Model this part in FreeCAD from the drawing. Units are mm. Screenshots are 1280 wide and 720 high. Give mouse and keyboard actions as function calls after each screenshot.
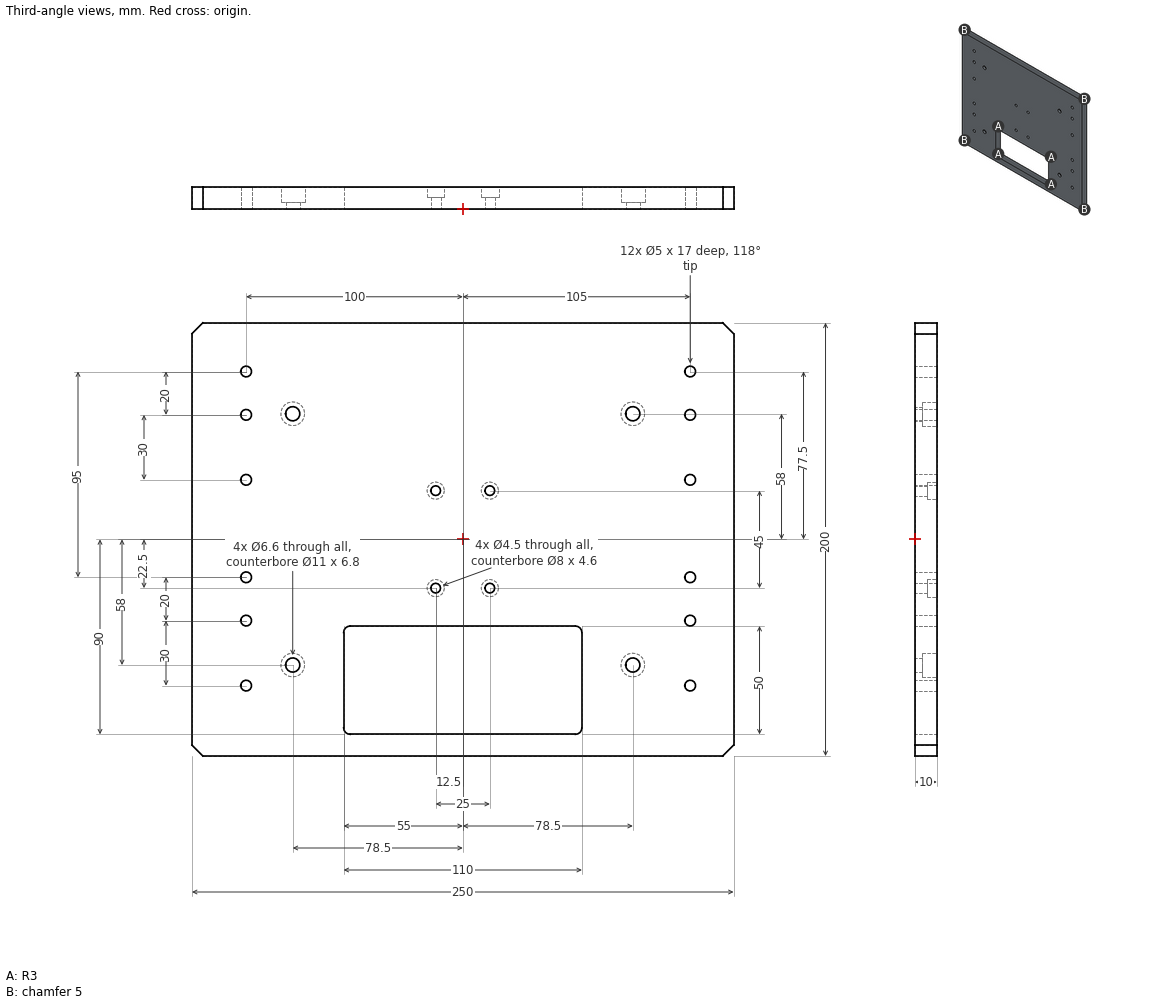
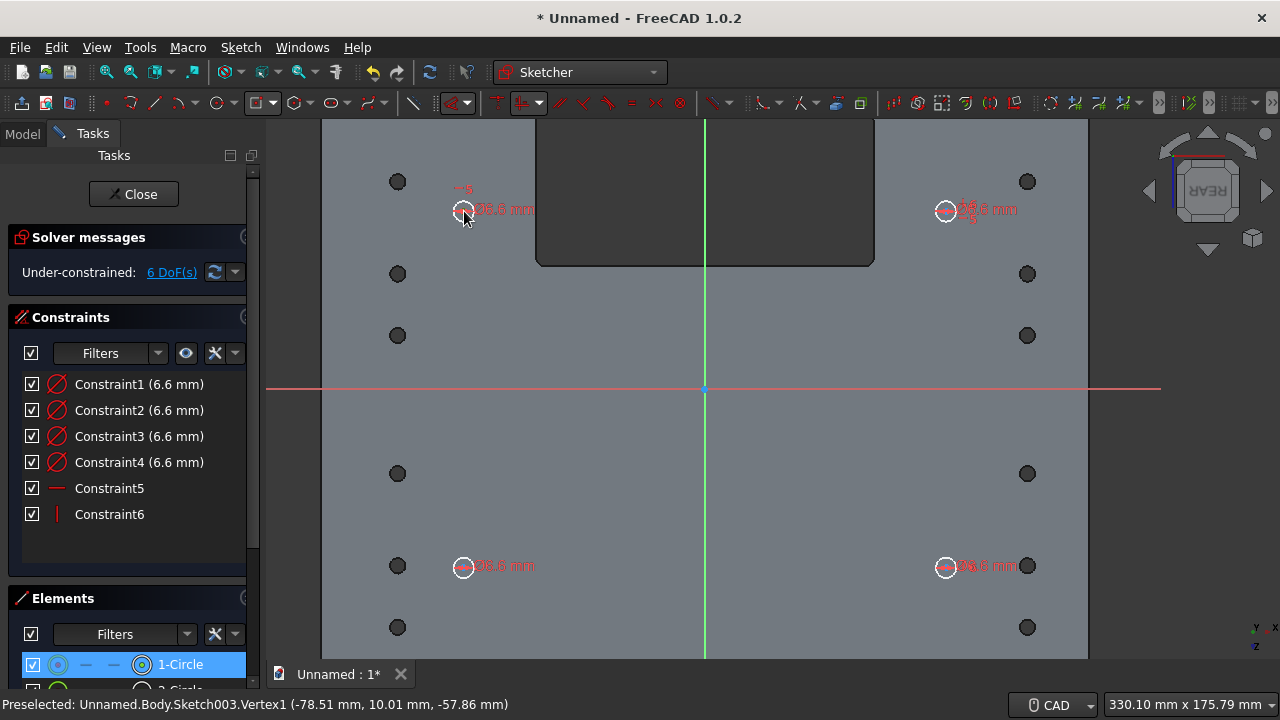
click(464, 568)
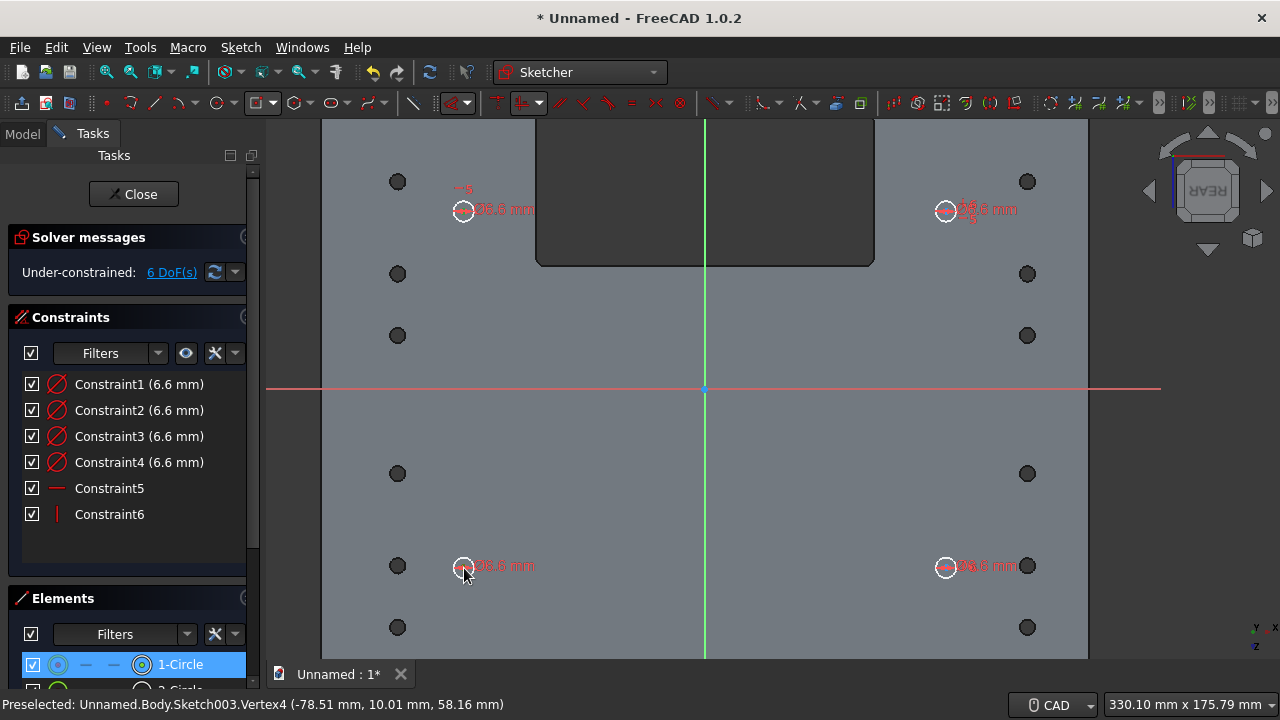
click(542, 104)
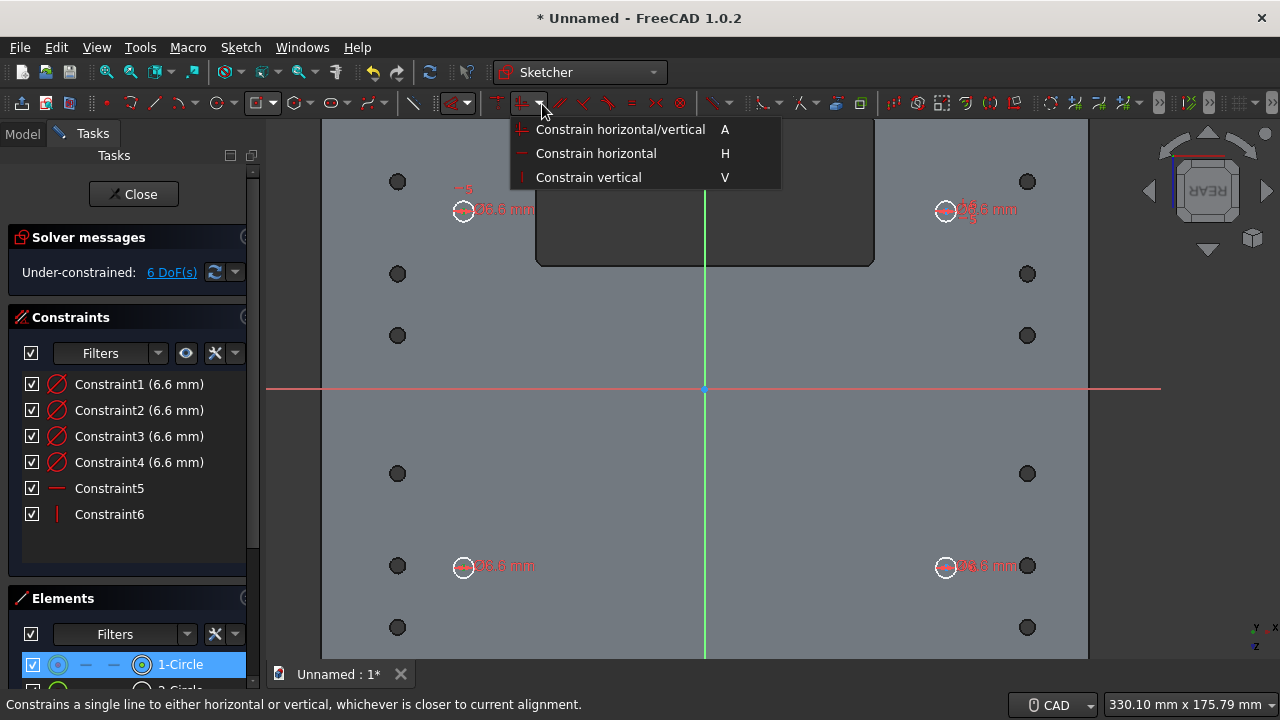
click(646, 177)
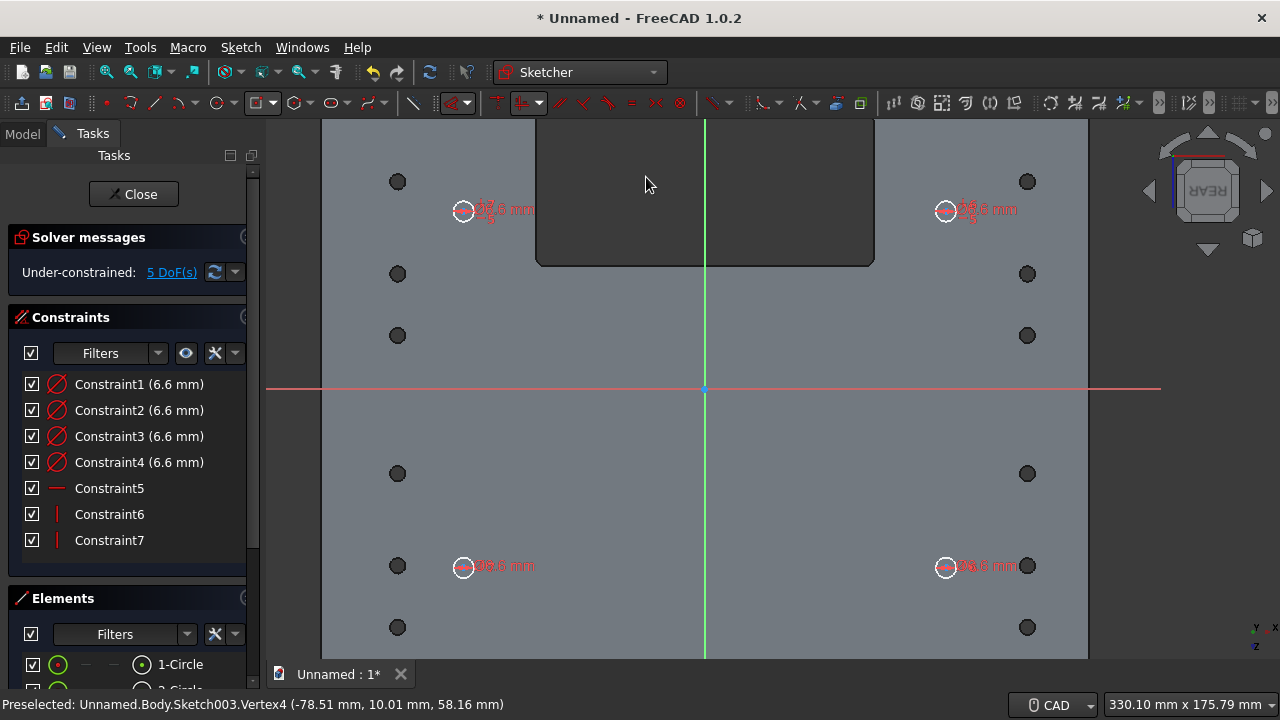
click(946, 568)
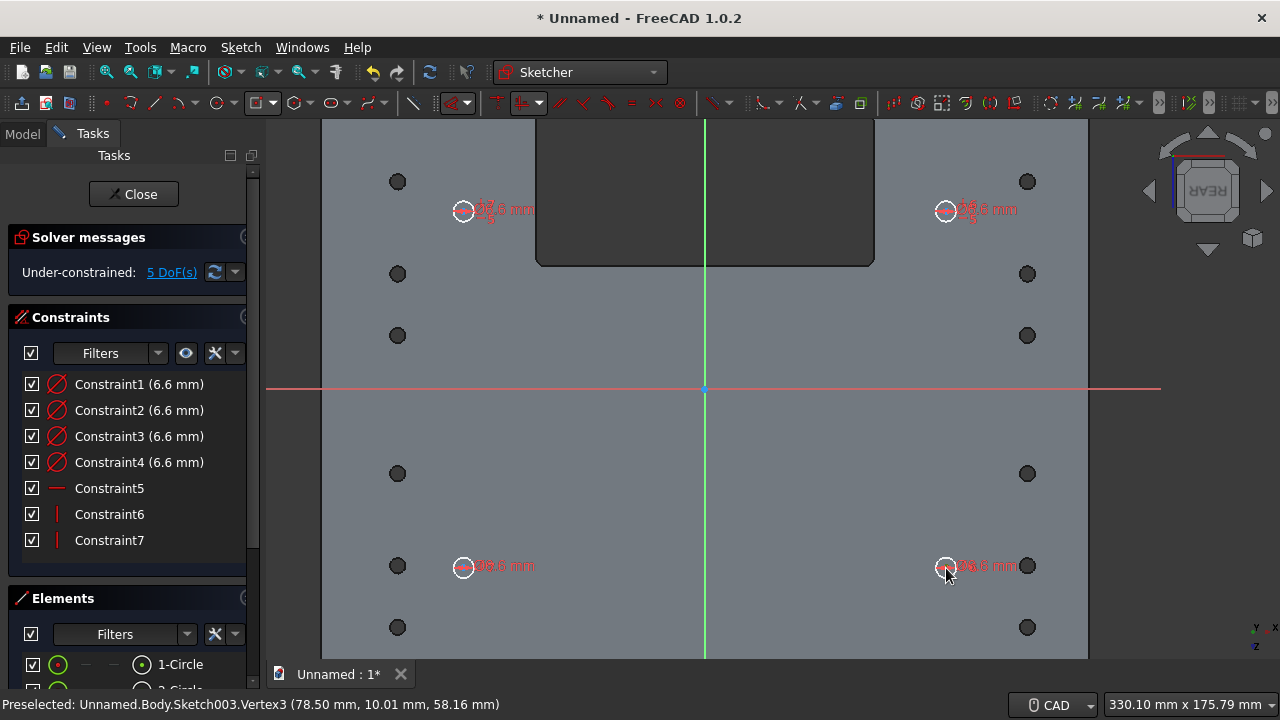
click(464, 568)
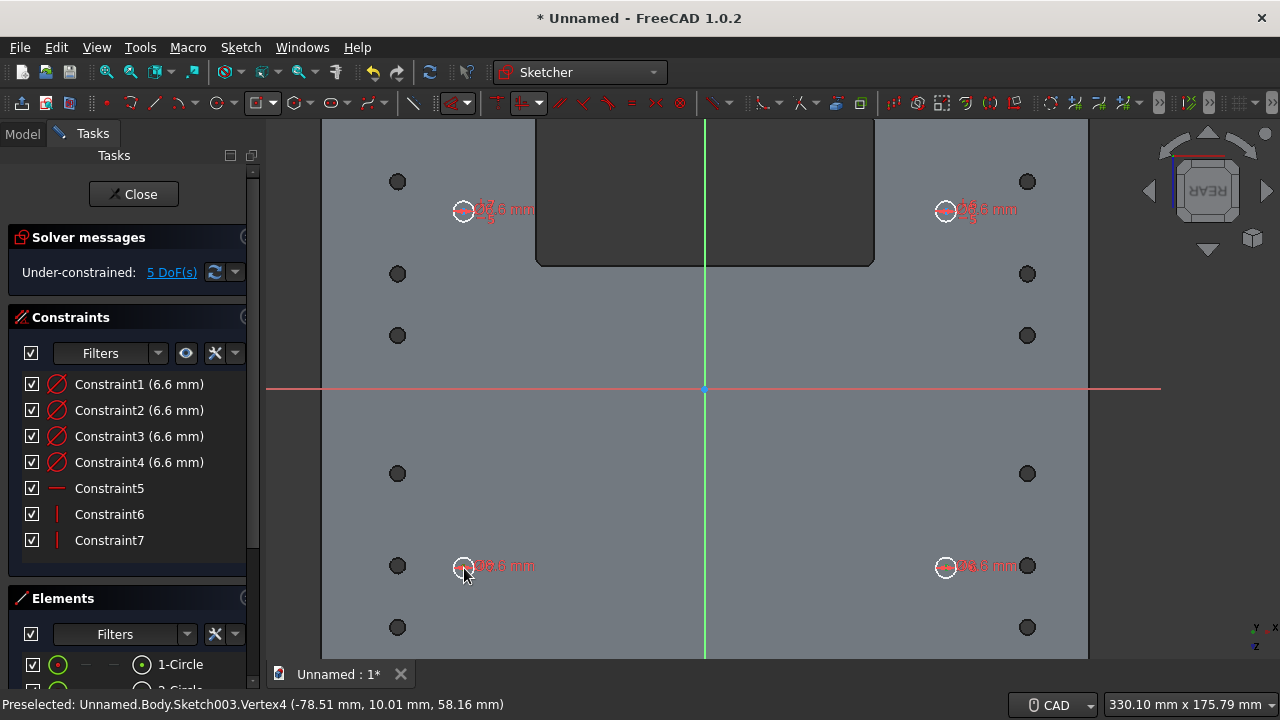
click(542, 104)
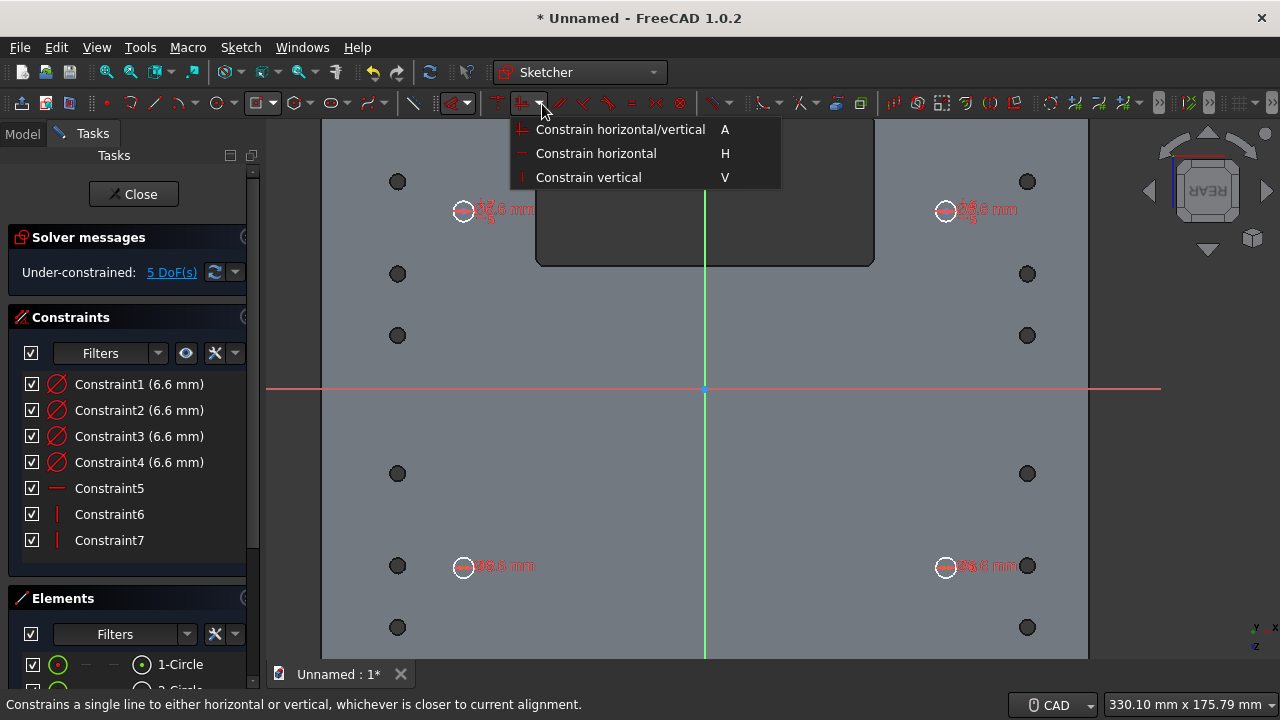
click(646, 153)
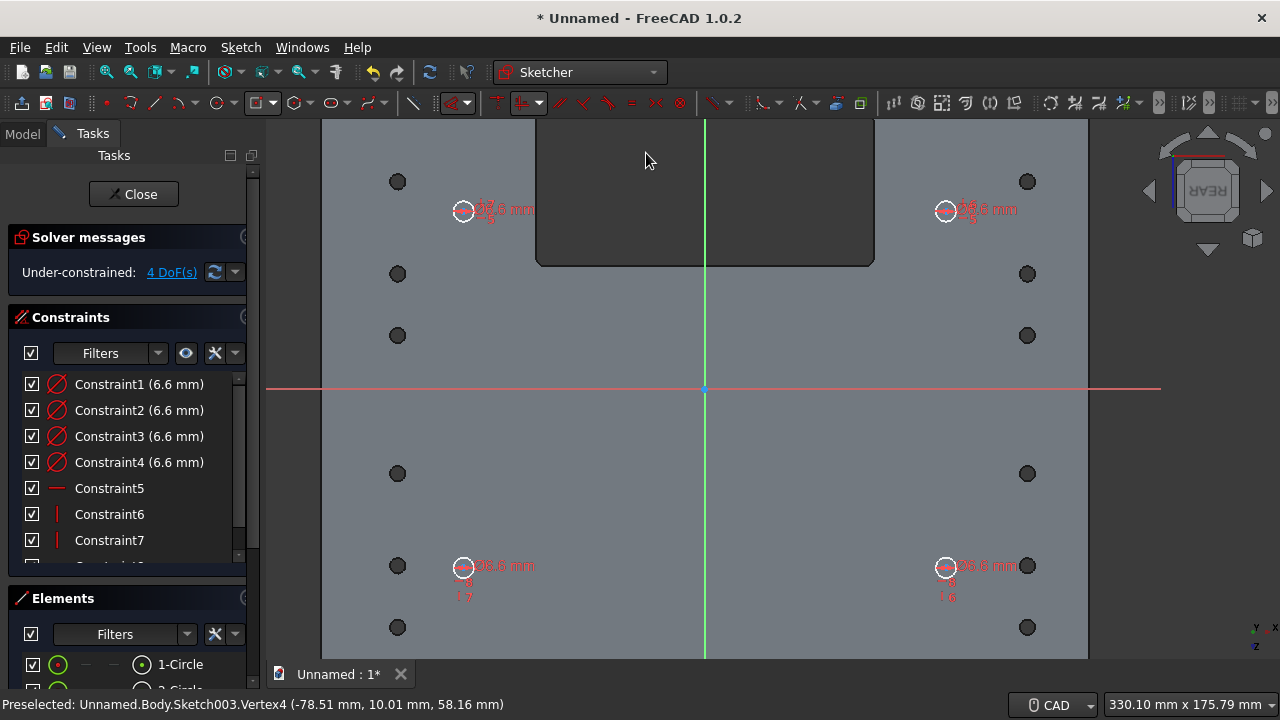
click(464, 211)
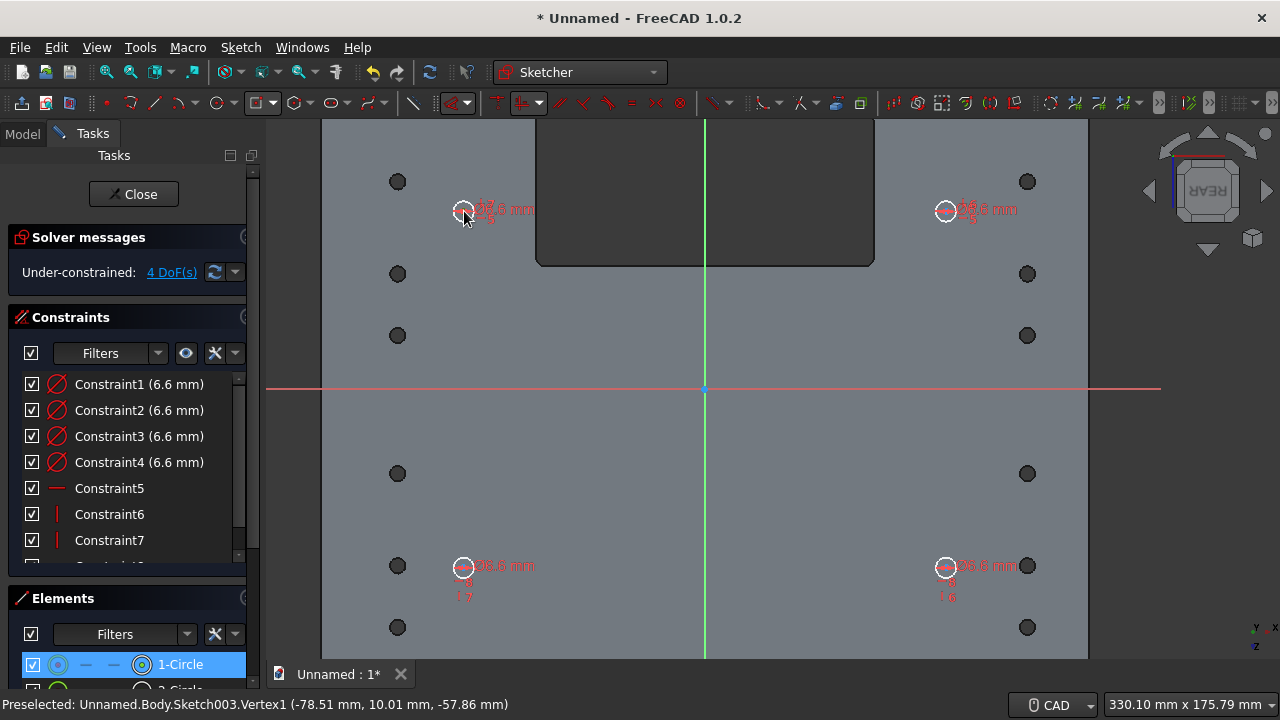
click(470, 104)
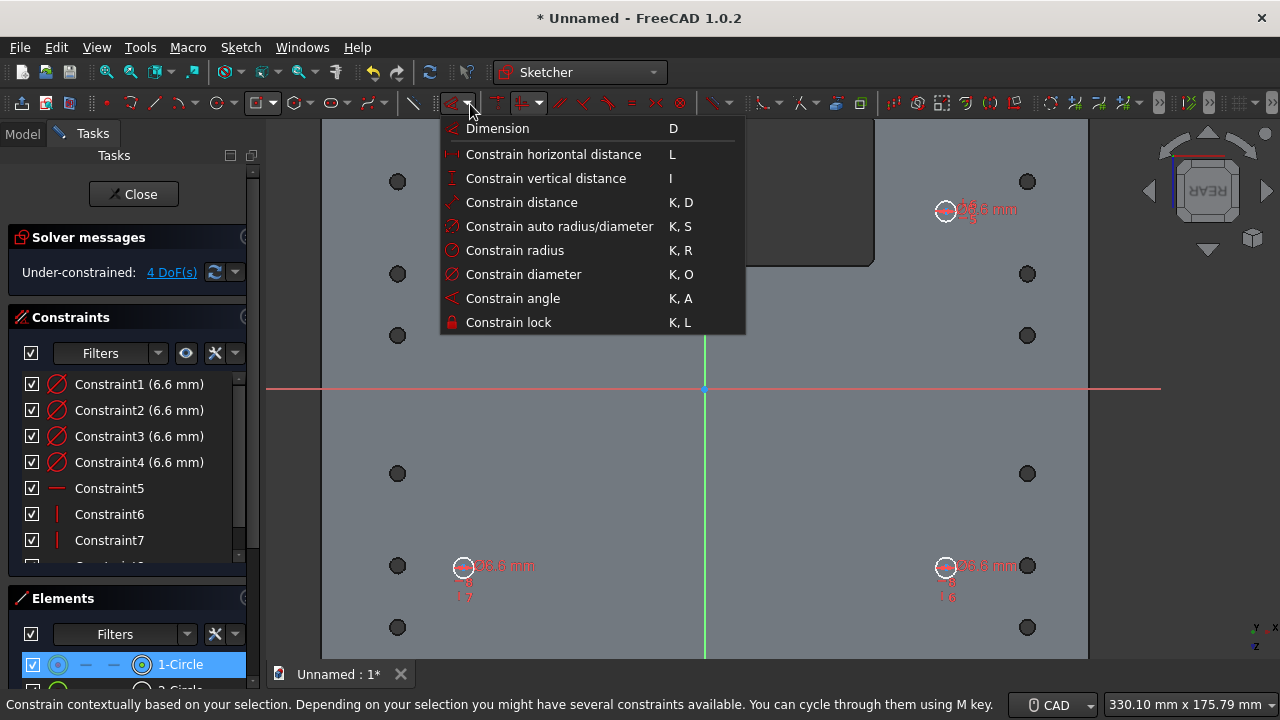
click(593, 178)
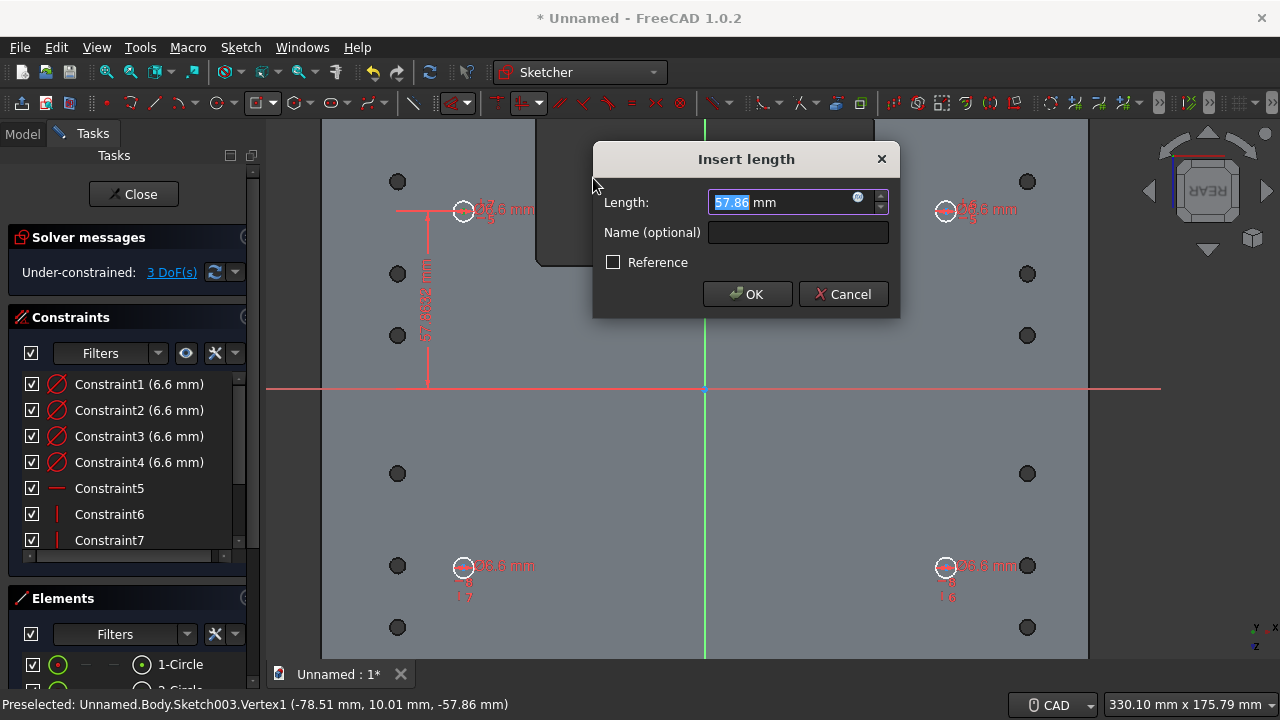
text(58)
key(Return)